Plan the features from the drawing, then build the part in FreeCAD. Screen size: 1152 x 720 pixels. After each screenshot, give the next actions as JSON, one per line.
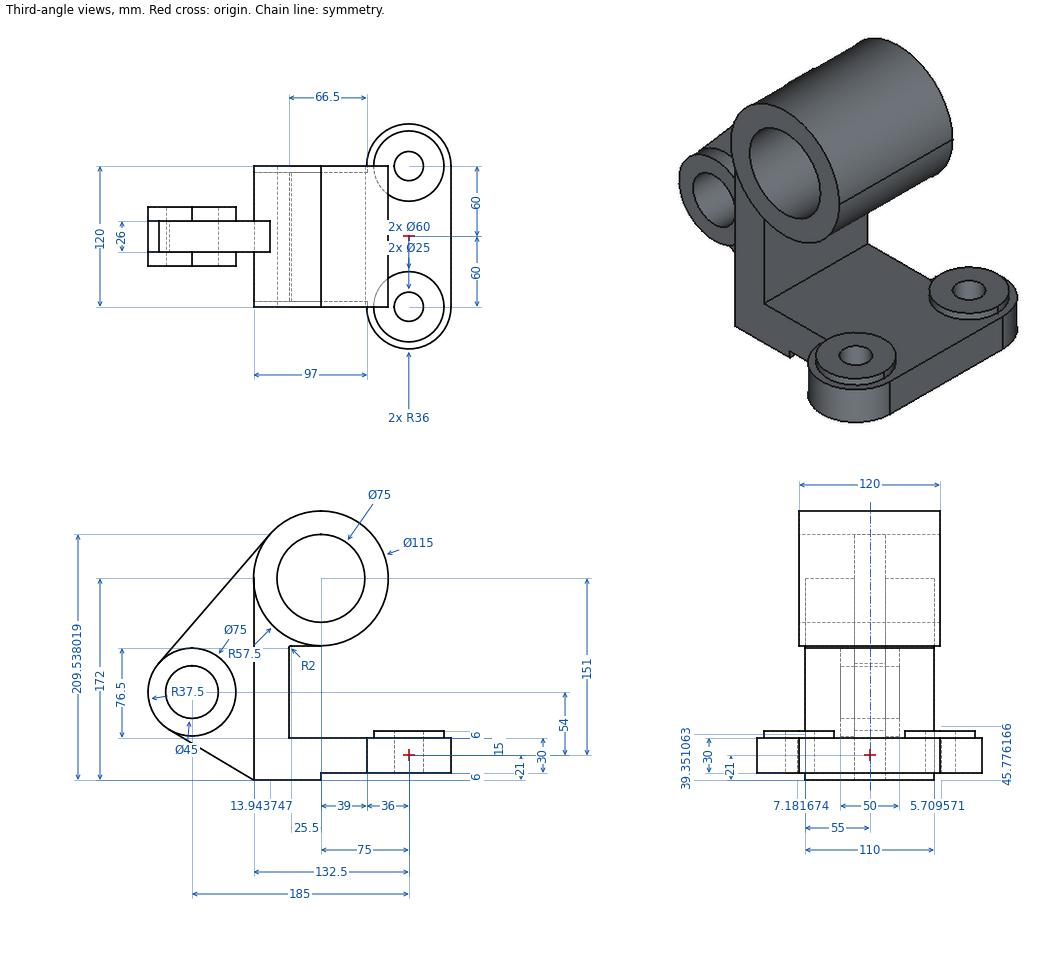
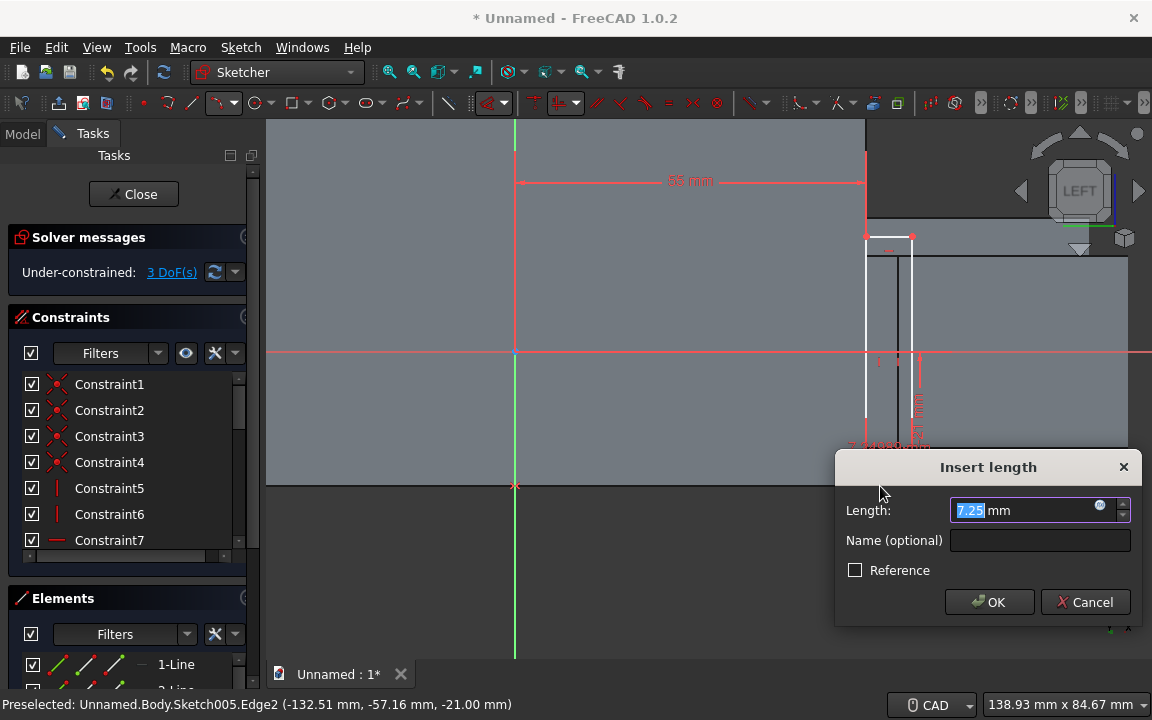
{"action": "type", "text": "7.181674"}
{"action": "key", "text": "Return"}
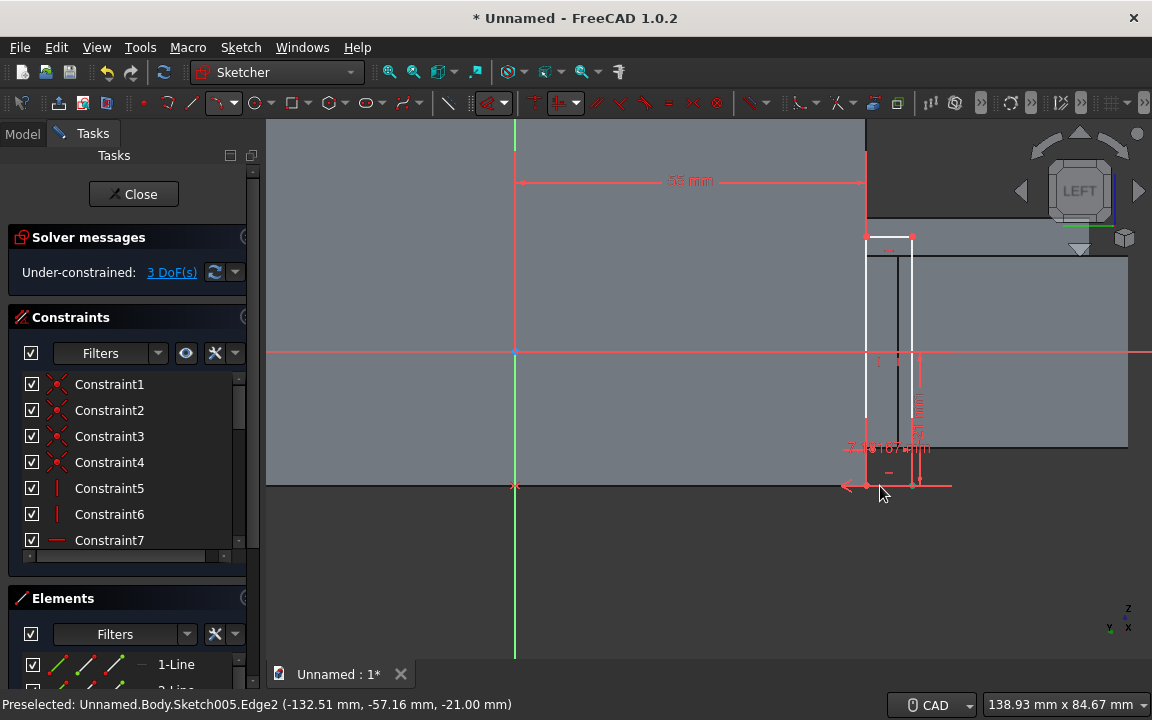
{"action": "scroll", "coordinate": [885, 489], "scroll_direction": "down", "scroll_amount": 2}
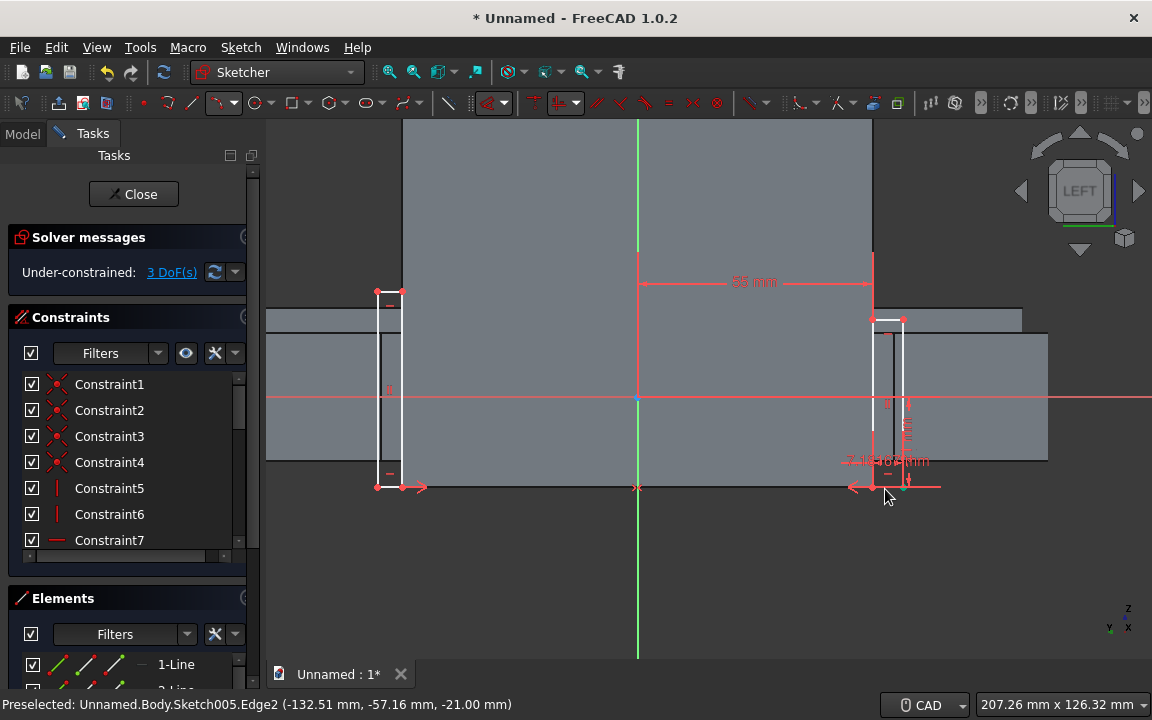
{"action": "scroll", "coordinate": [385, 487], "scroll_direction": "up", "scroll_amount": 4}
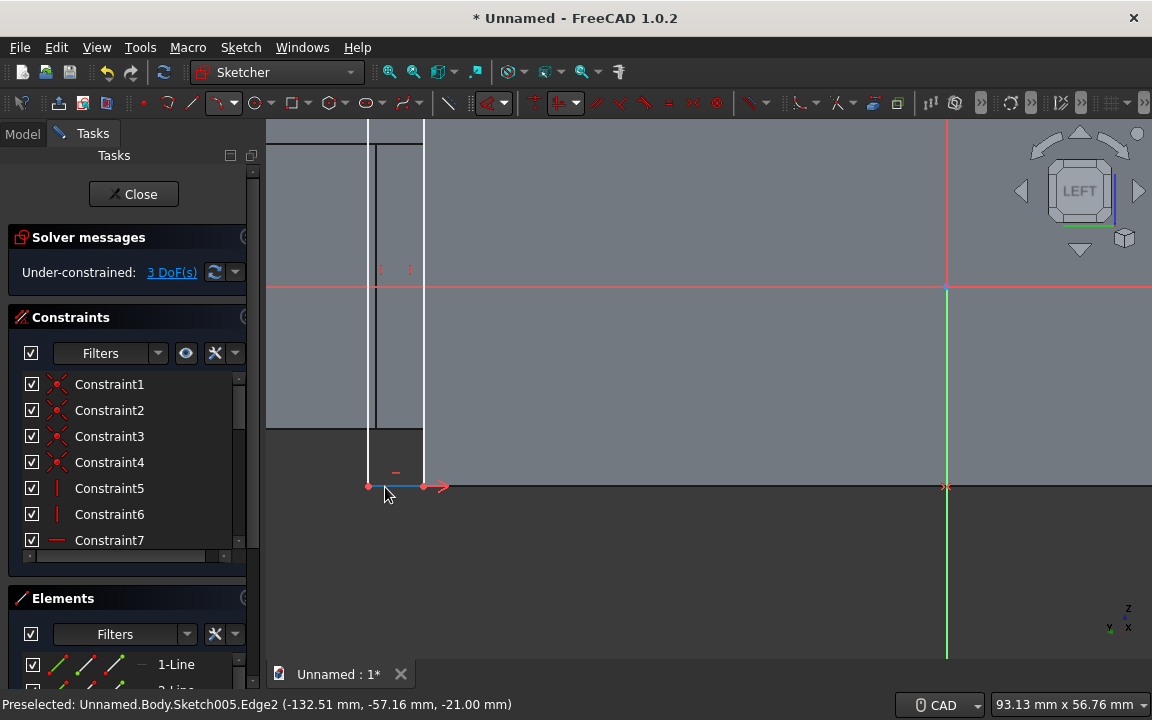
{"action": "left_click", "coordinate": [385, 486]}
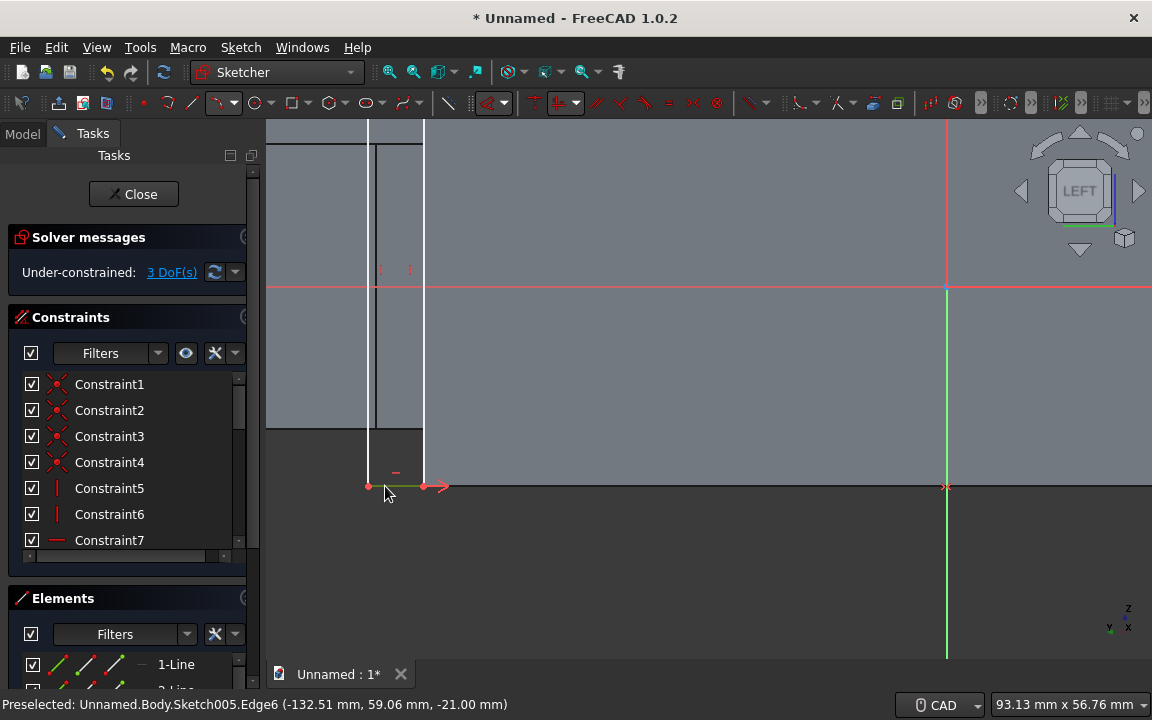
{"action": "key", "text": "l"}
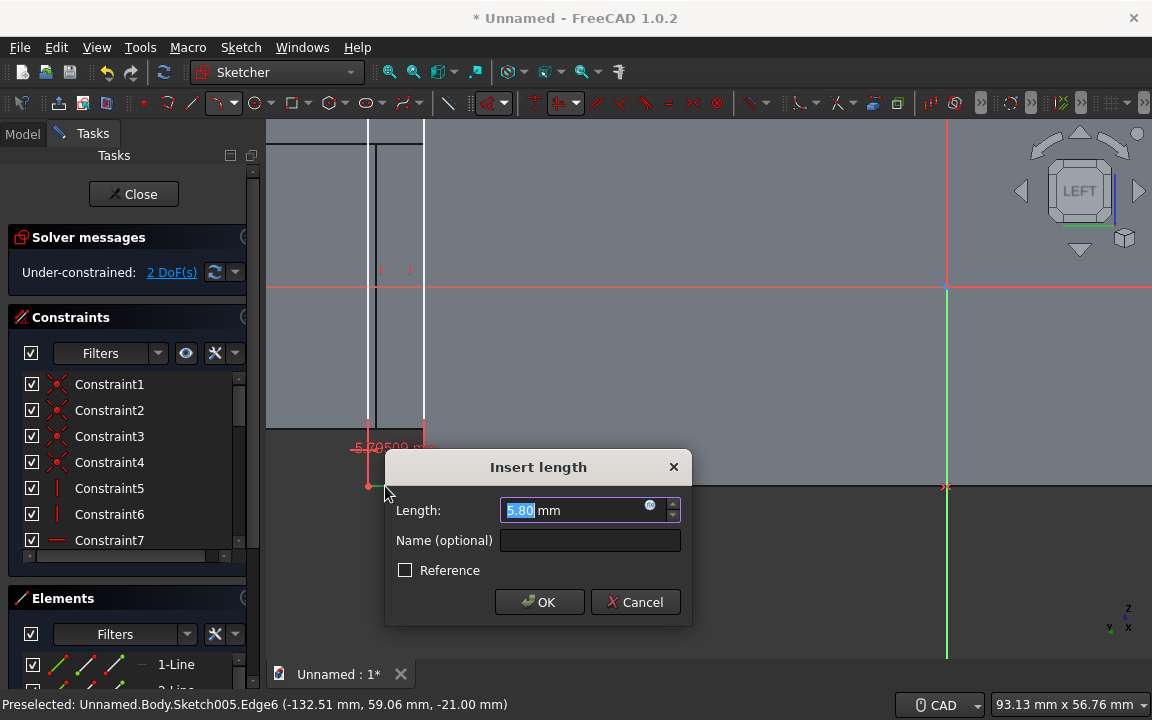
{"action": "type", "text": "5.709571"}
{"action": "key", "text": "Return"}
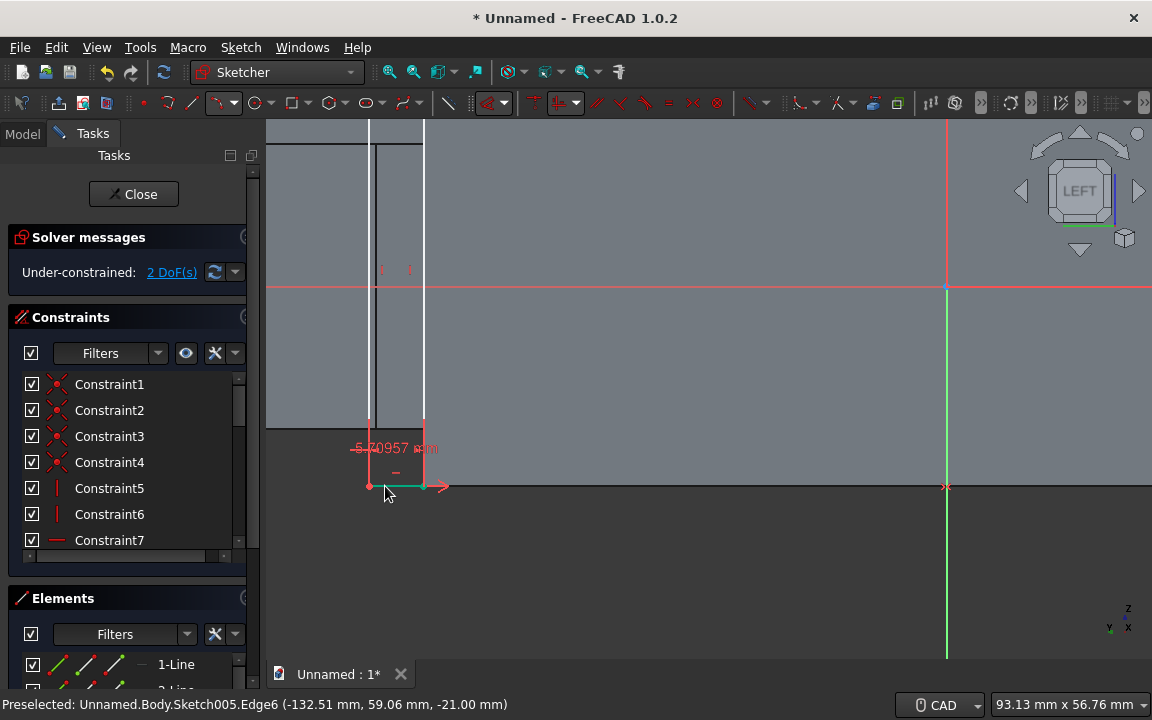
{"action": "scroll", "coordinate": [385, 487], "scroll_direction": "down", "scroll_amount": 4}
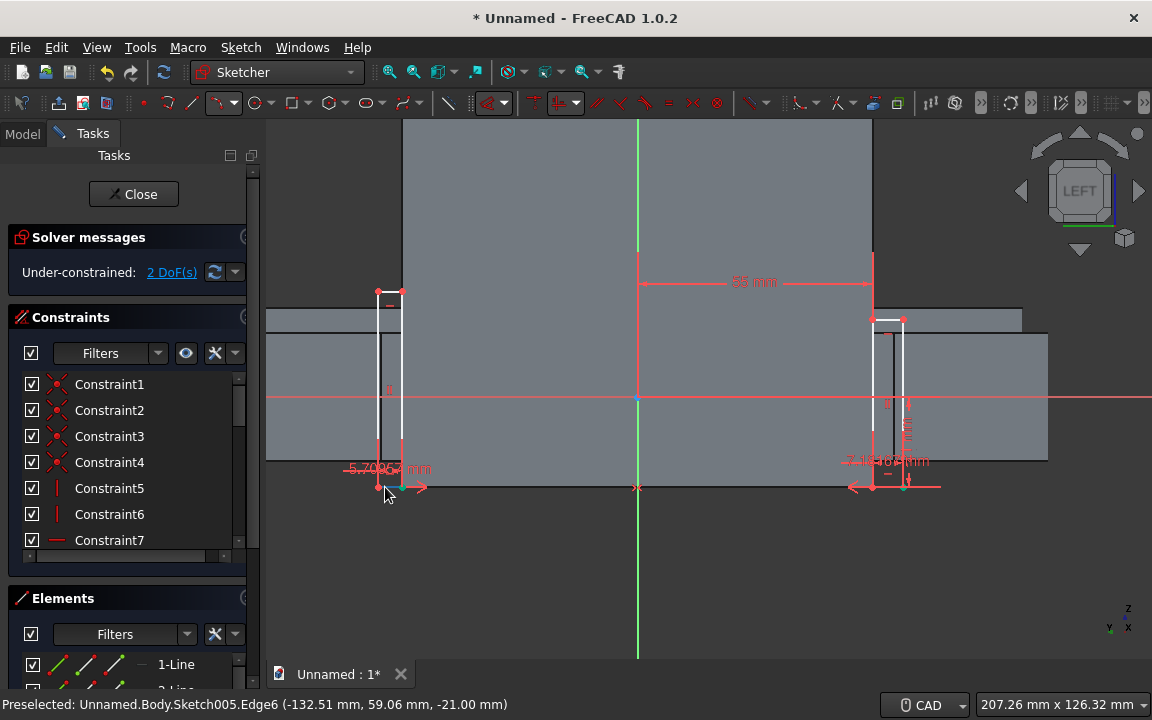
{"action": "left_click", "coordinate": [873, 370]}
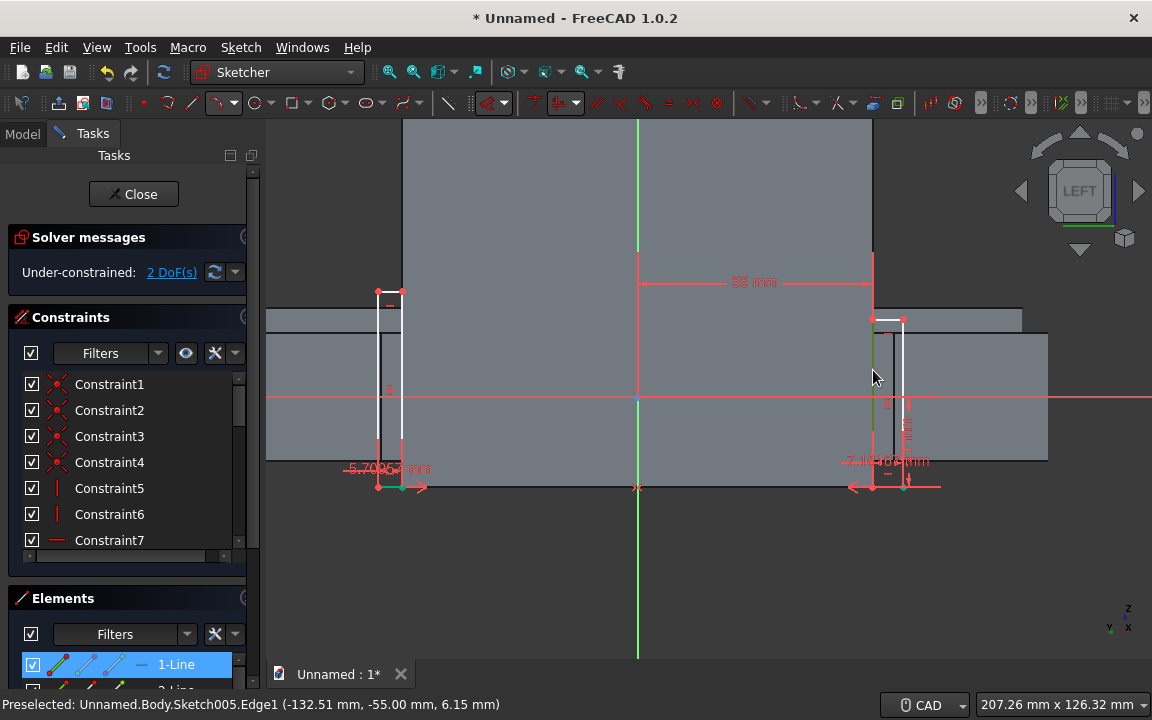
{"action": "key", "text": "i"}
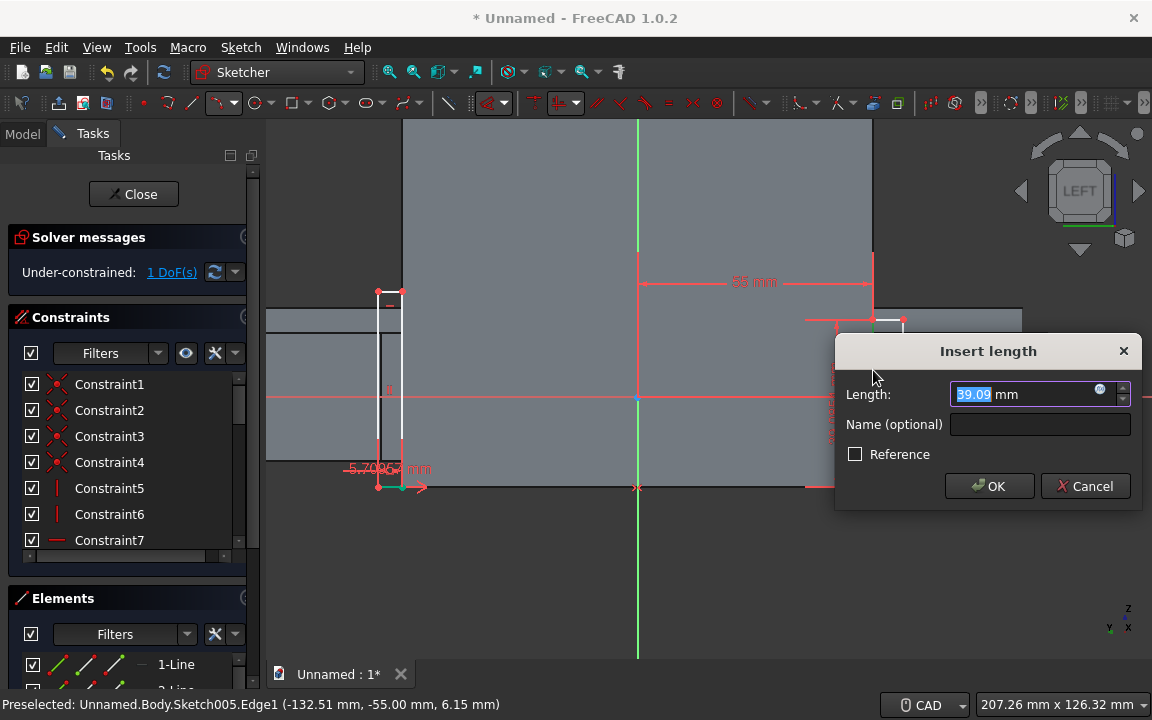
{"action": "type", "text": "39.351063"}
{"action": "key", "text": "Return"}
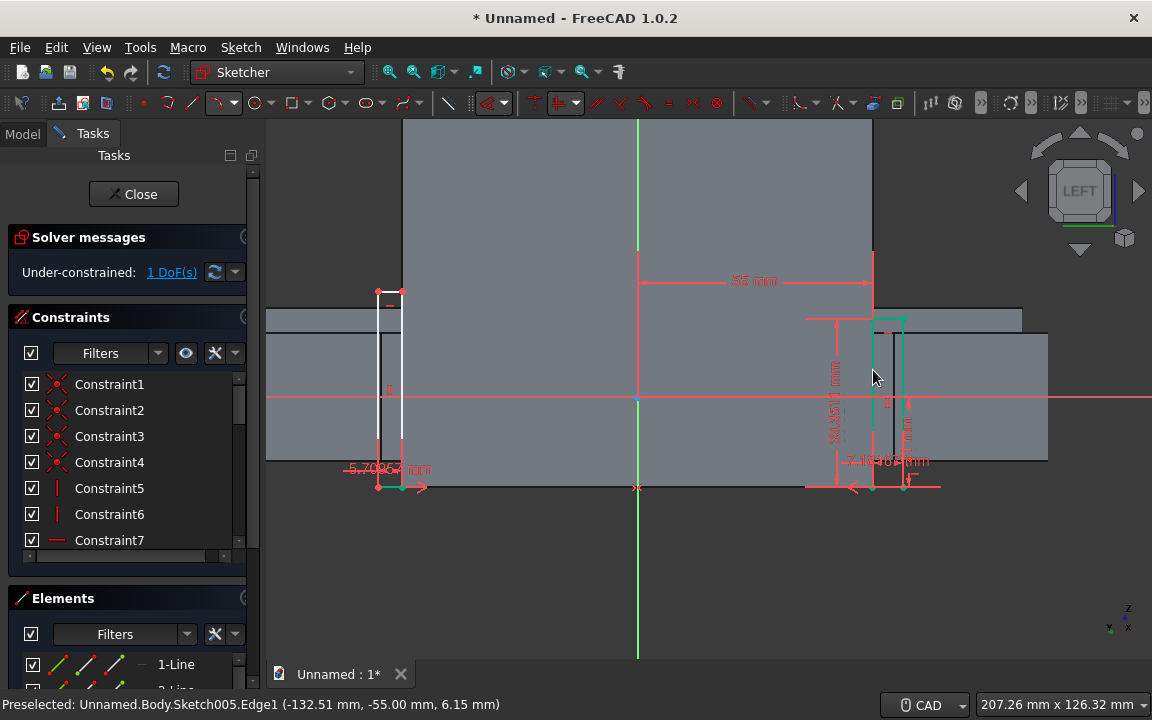
{"action": "left_click", "coordinate": [378, 351]}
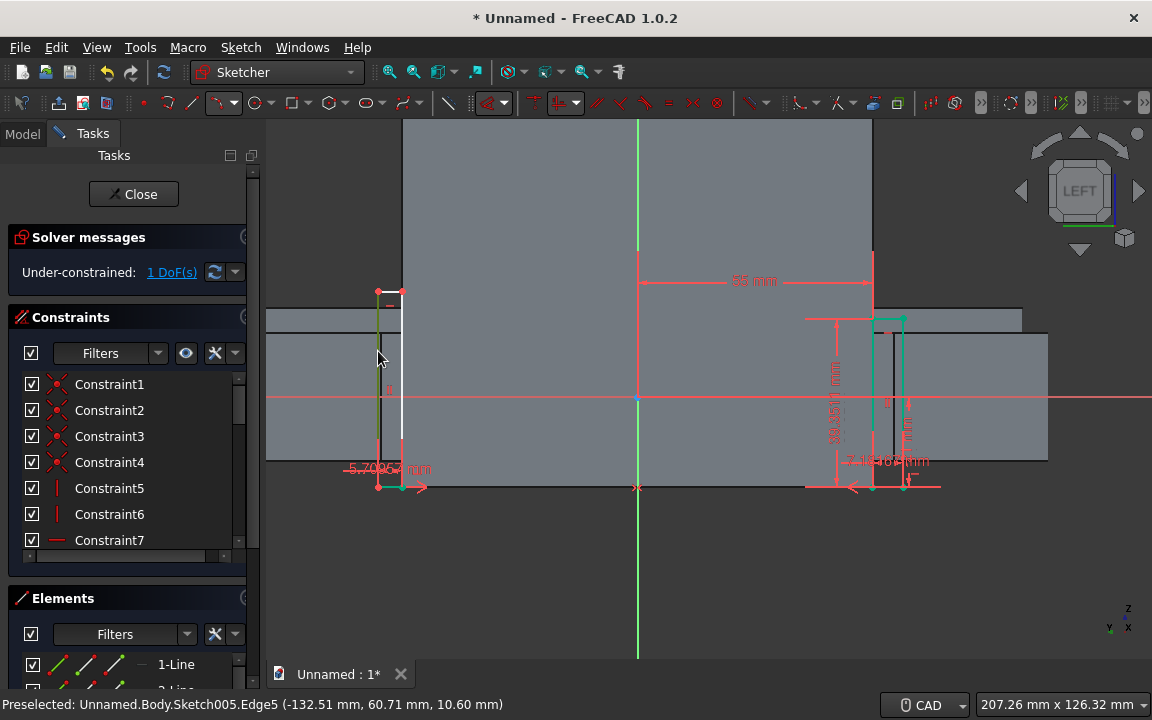
{"action": "key", "text": "i"}